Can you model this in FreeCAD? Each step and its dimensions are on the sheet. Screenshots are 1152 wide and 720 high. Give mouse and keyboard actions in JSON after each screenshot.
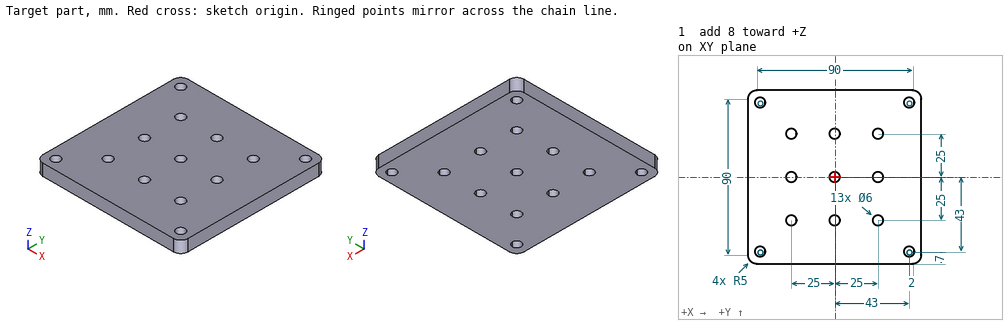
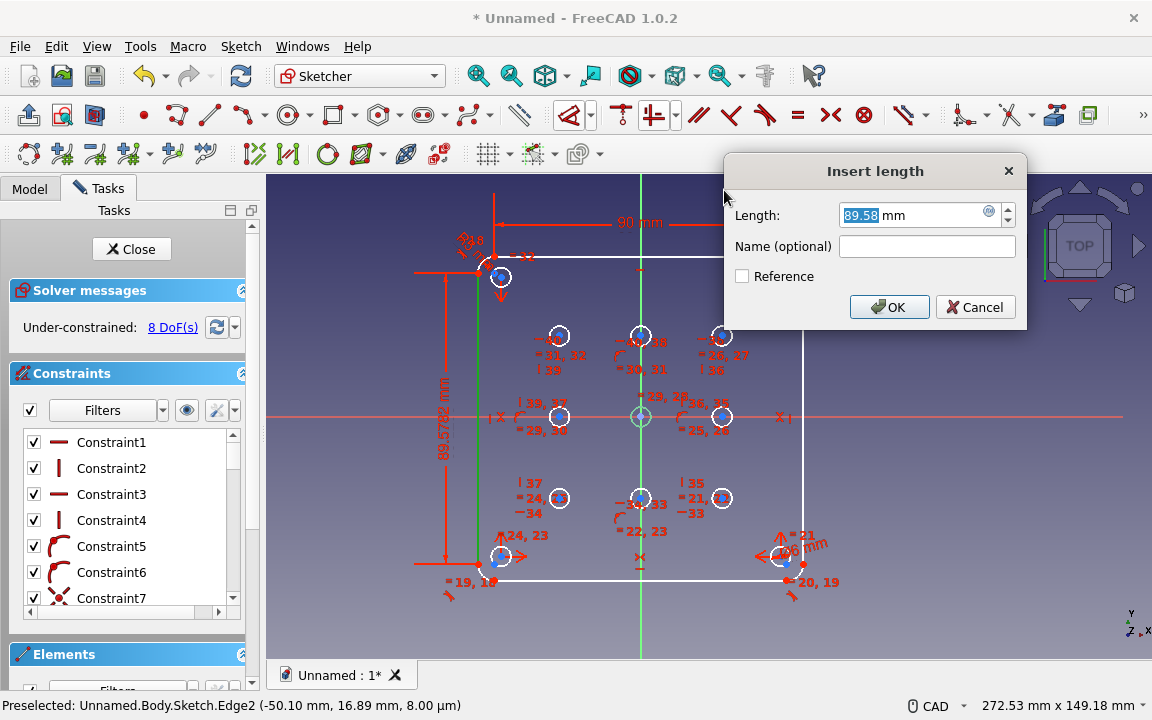
{"action": "type", "text": "90"}
{"action": "key", "text": "Return"}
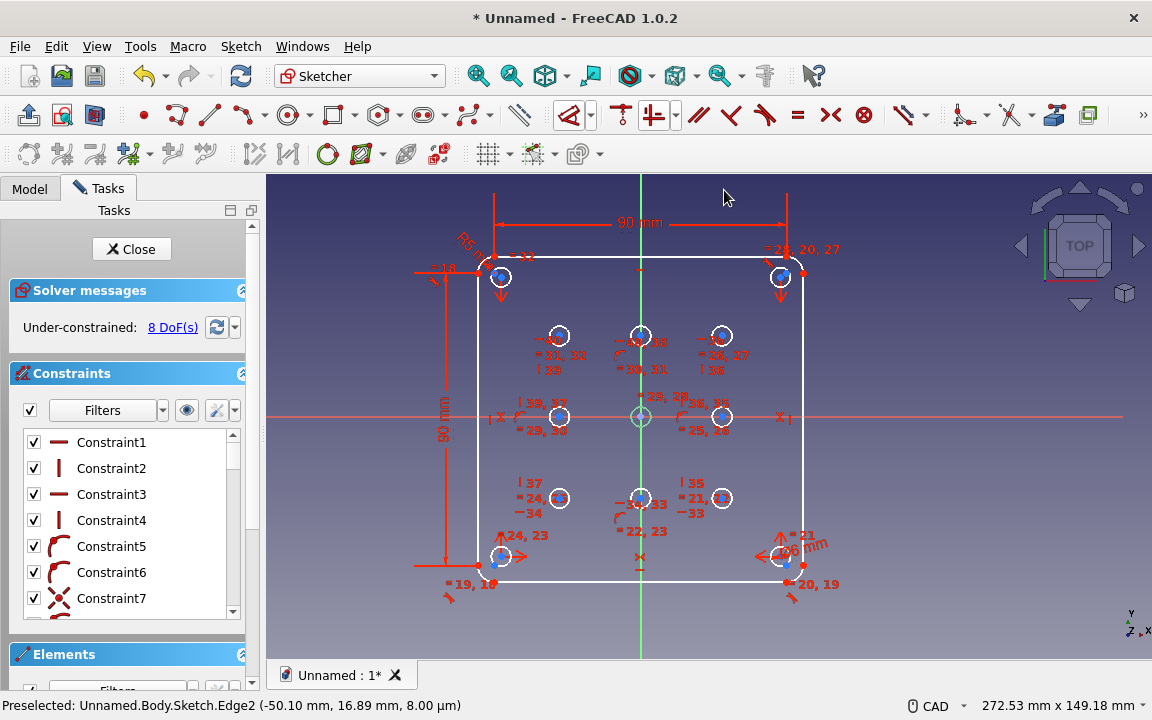
{"action": "left_click", "coordinate": [781, 556]}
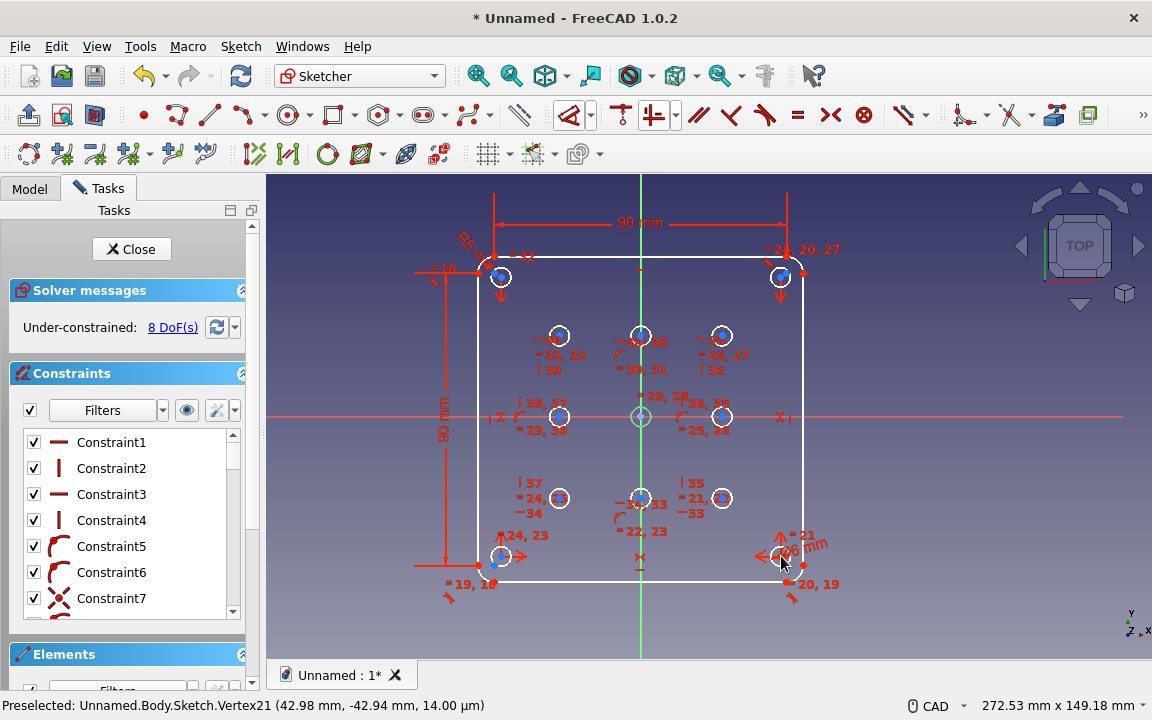
{"action": "key", "text": "l"}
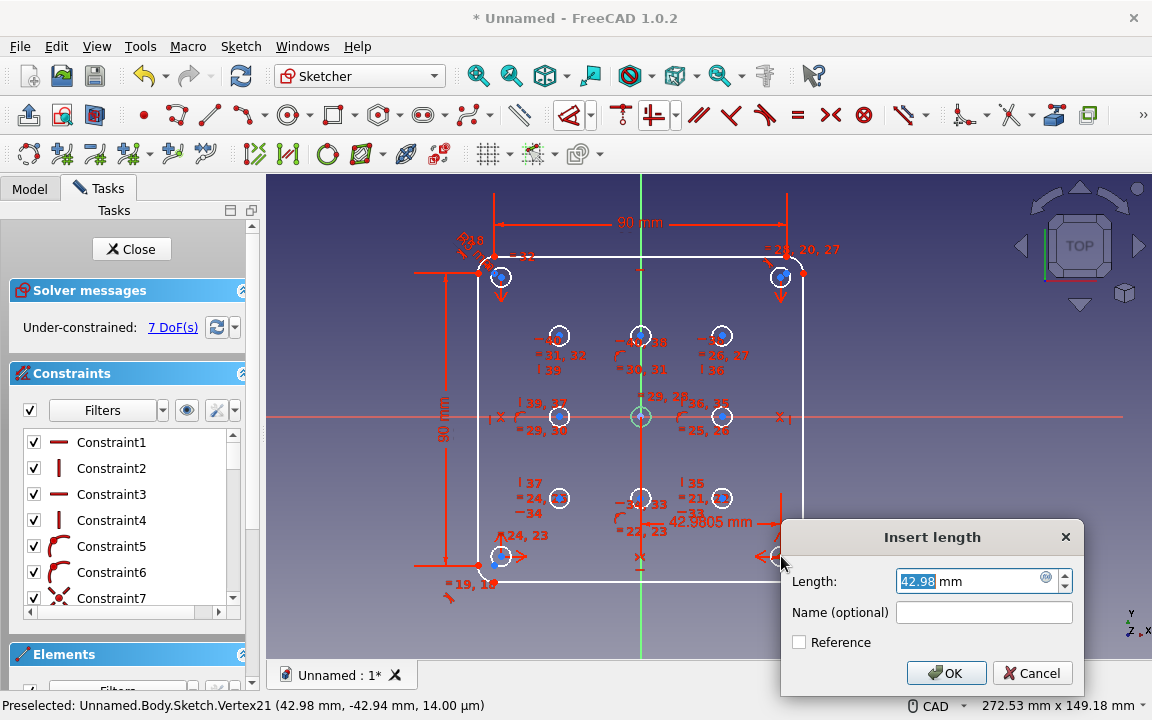
{"action": "type", "text": "43"}
{"action": "key", "text": "Return"}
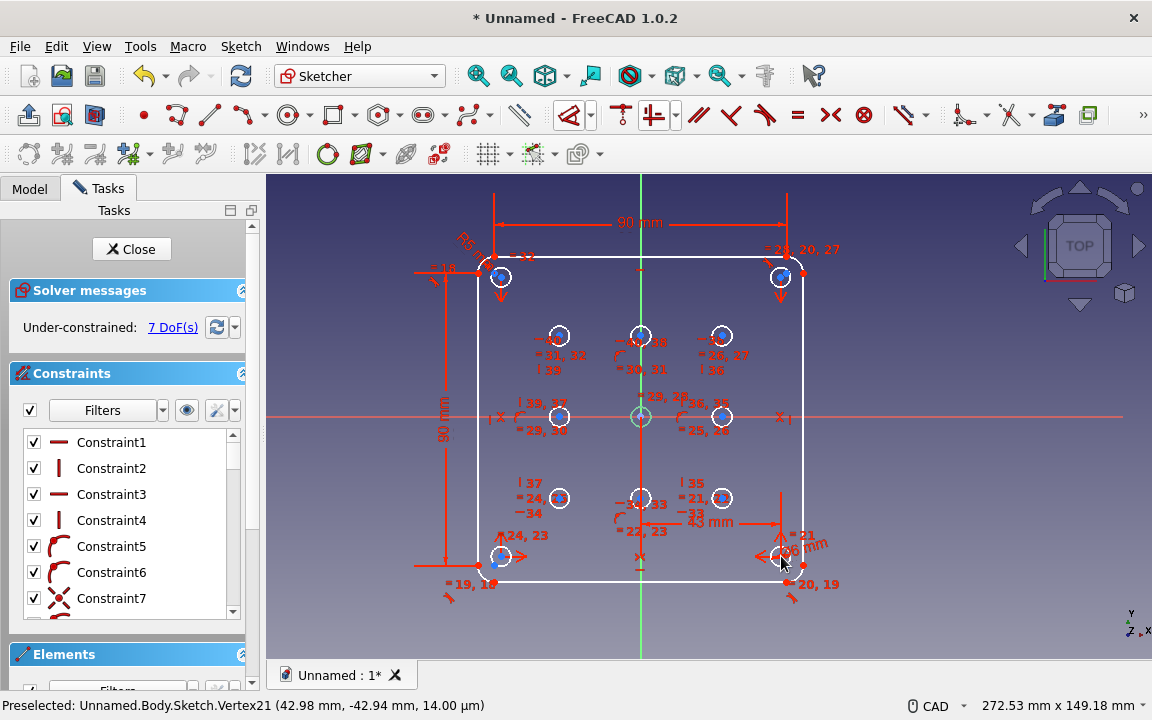
{"action": "left_click", "coordinate": [781, 556]}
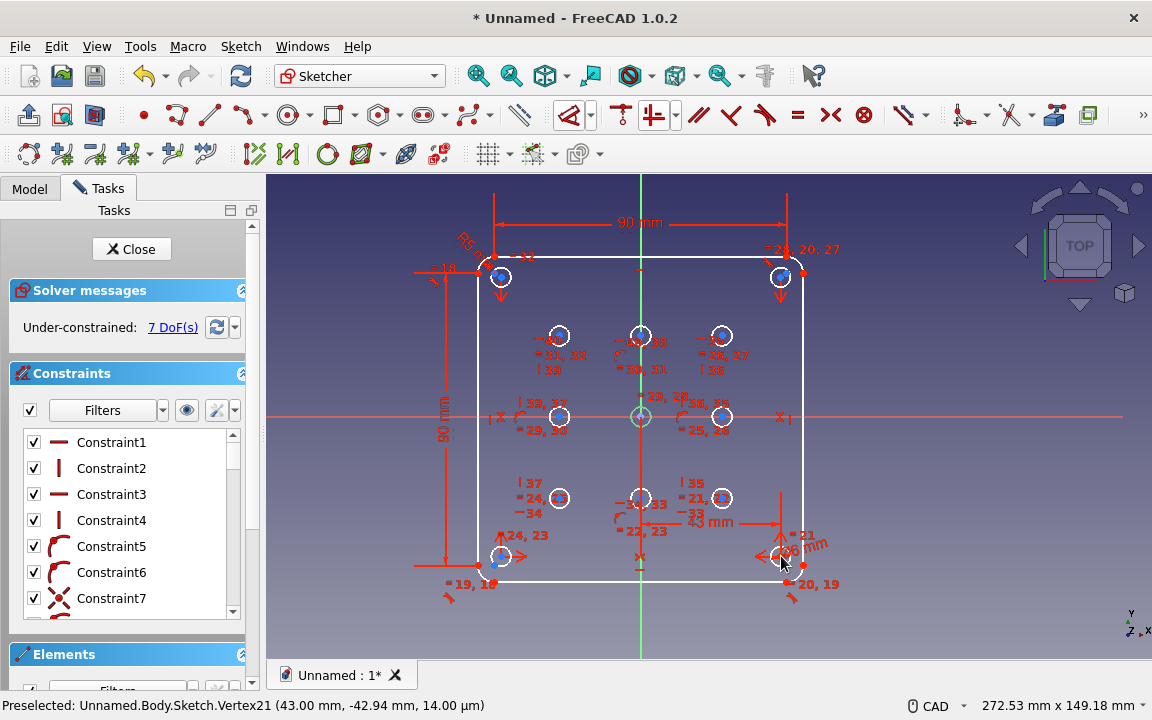
{"action": "left_click", "coordinate": [590, 116]}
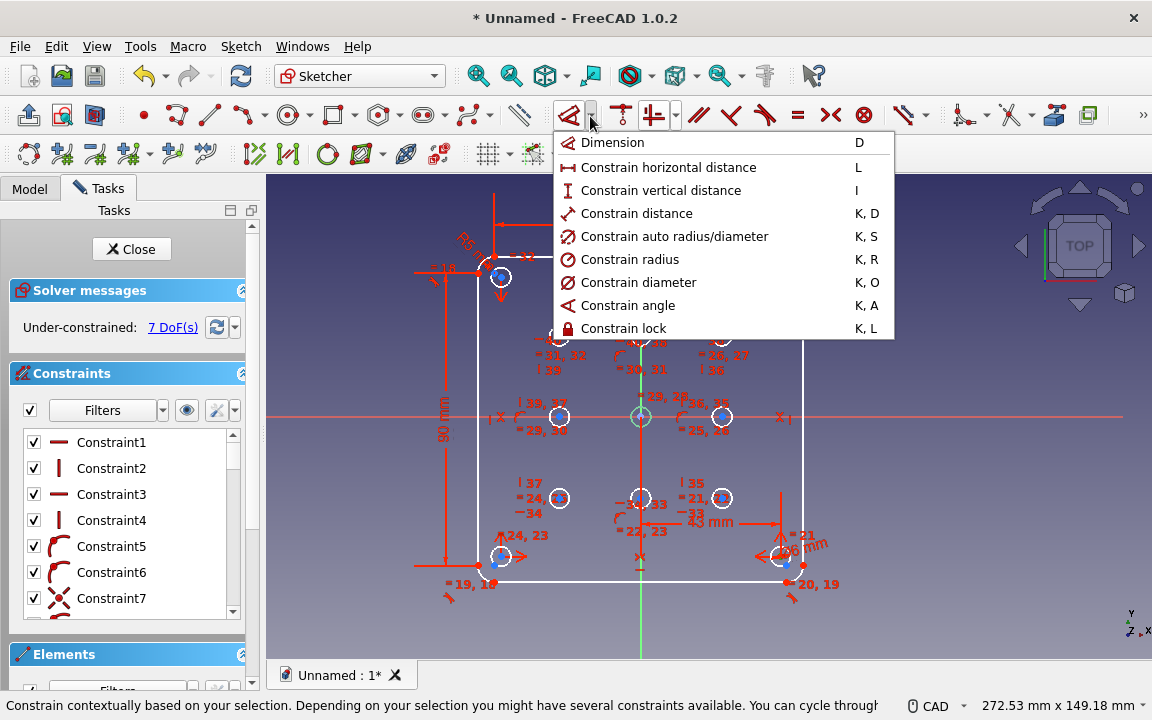
{"action": "left_click", "coordinate": [724, 190]}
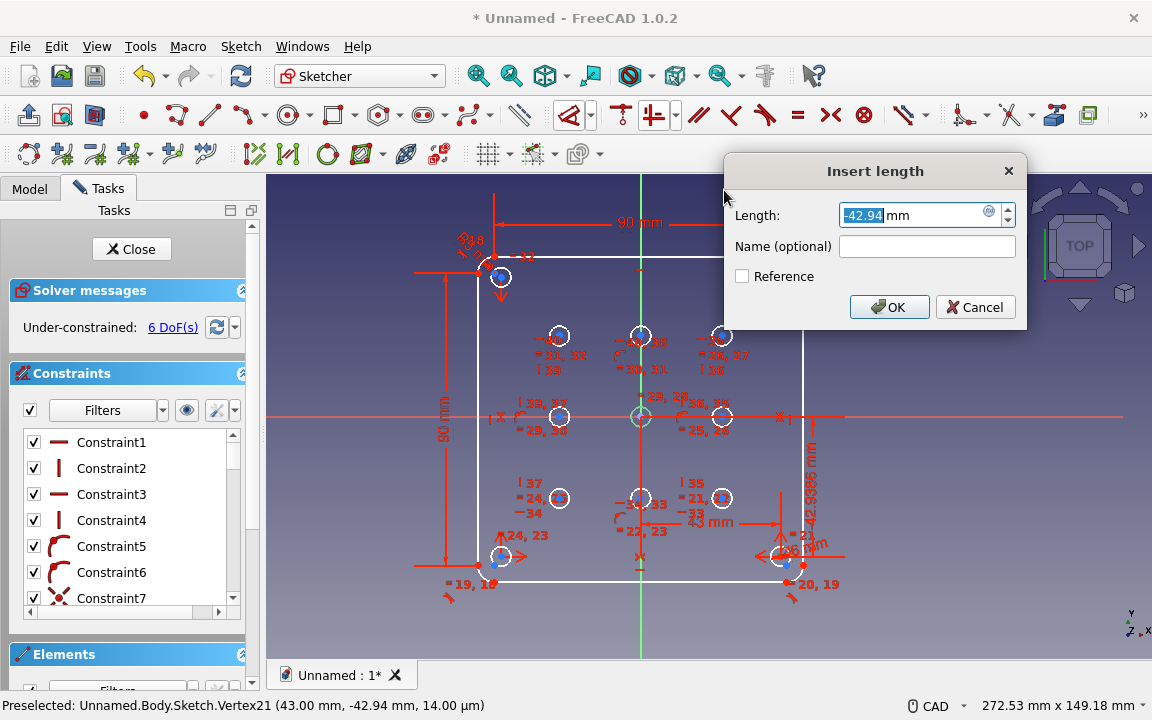
{"action": "type", "text": "-43"}
{"action": "key", "text": "Return"}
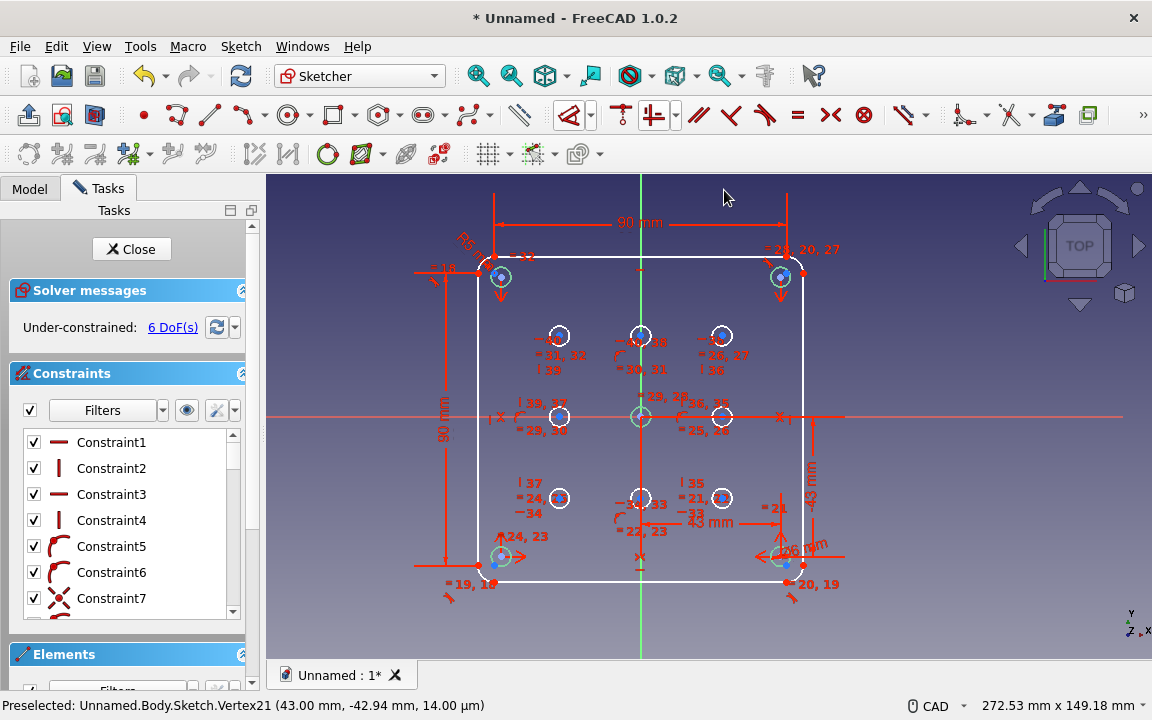
{"action": "left_click", "coordinate": [722, 498]}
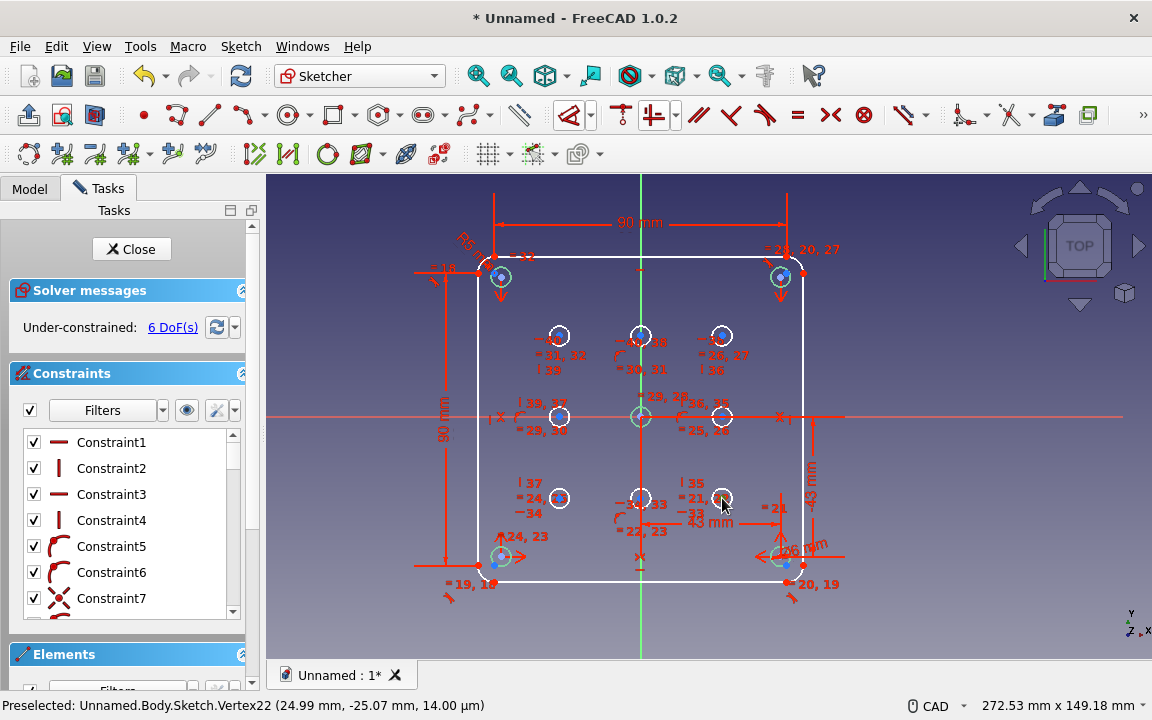
{"action": "left_click", "coordinate": [590, 116]}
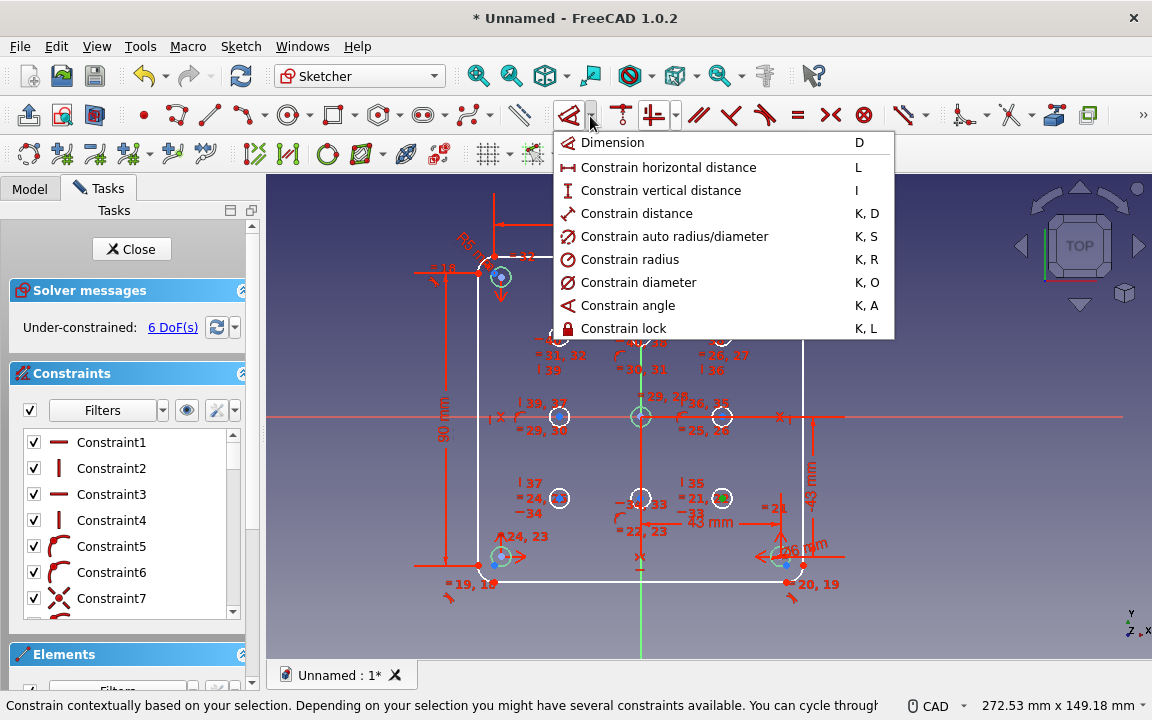
{"action": "left_click", "coordinate": [724, 168]}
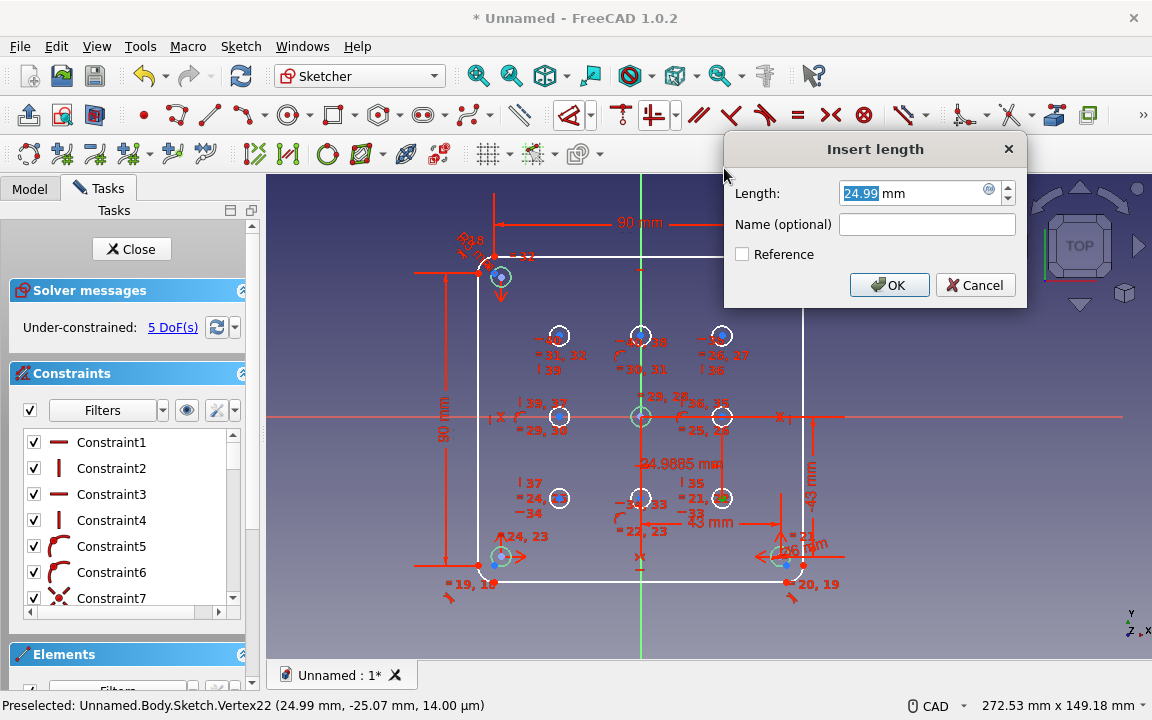
{"action": "type", "text": "25"}
{"action": "key", "text": "Return"}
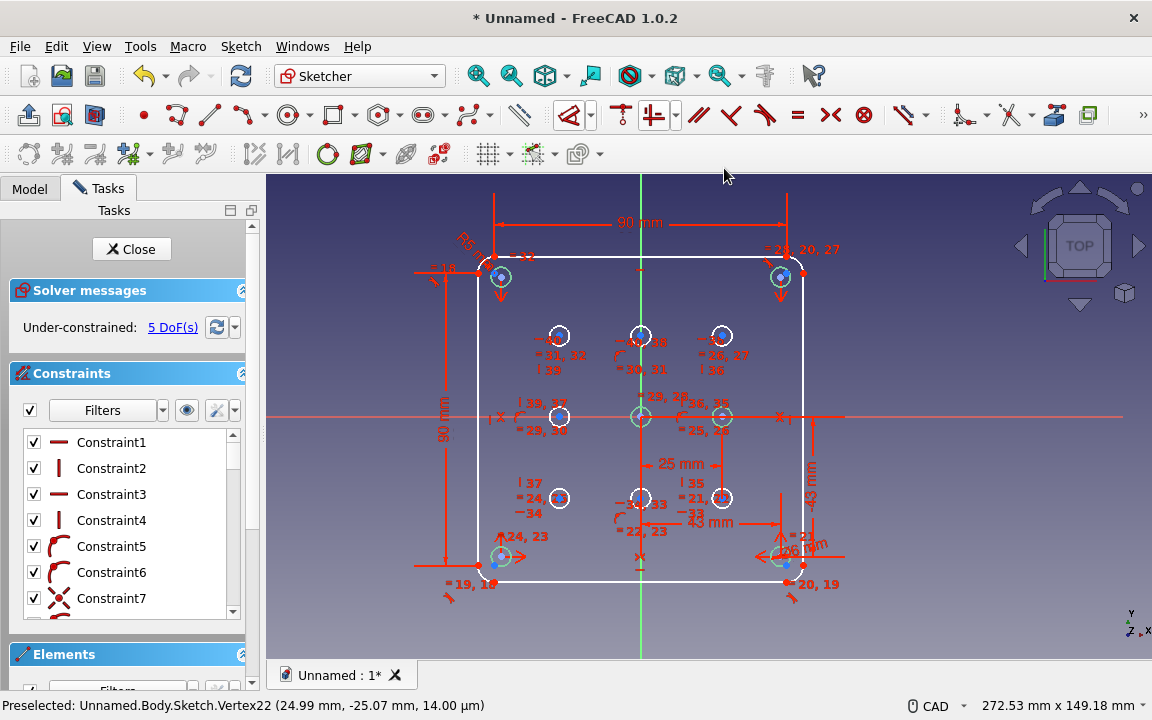
{"action": "left_click", "coordinate": [722, 498]}